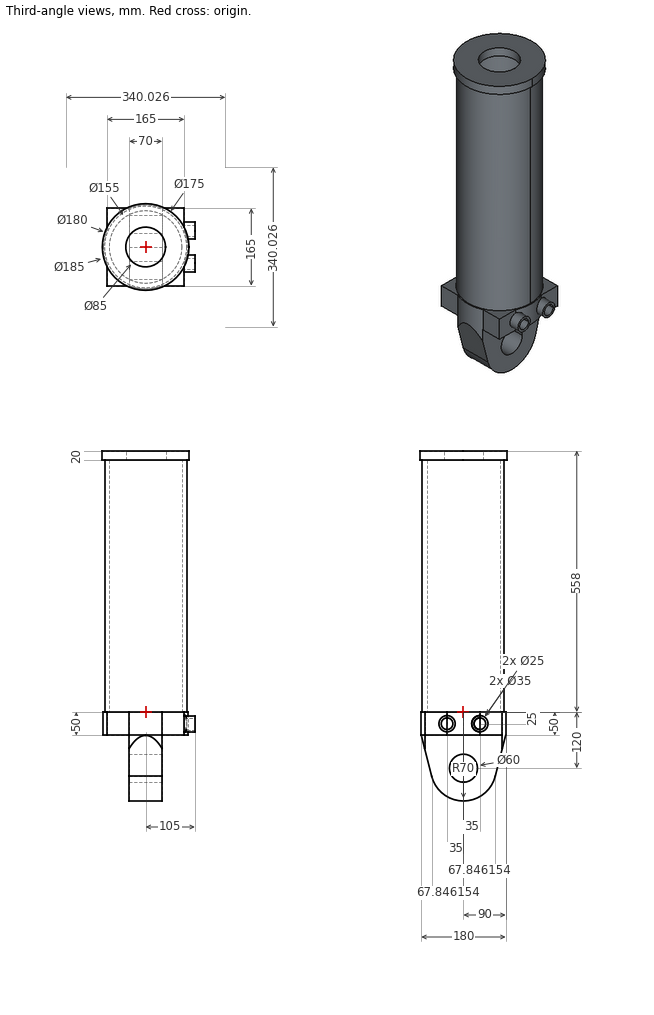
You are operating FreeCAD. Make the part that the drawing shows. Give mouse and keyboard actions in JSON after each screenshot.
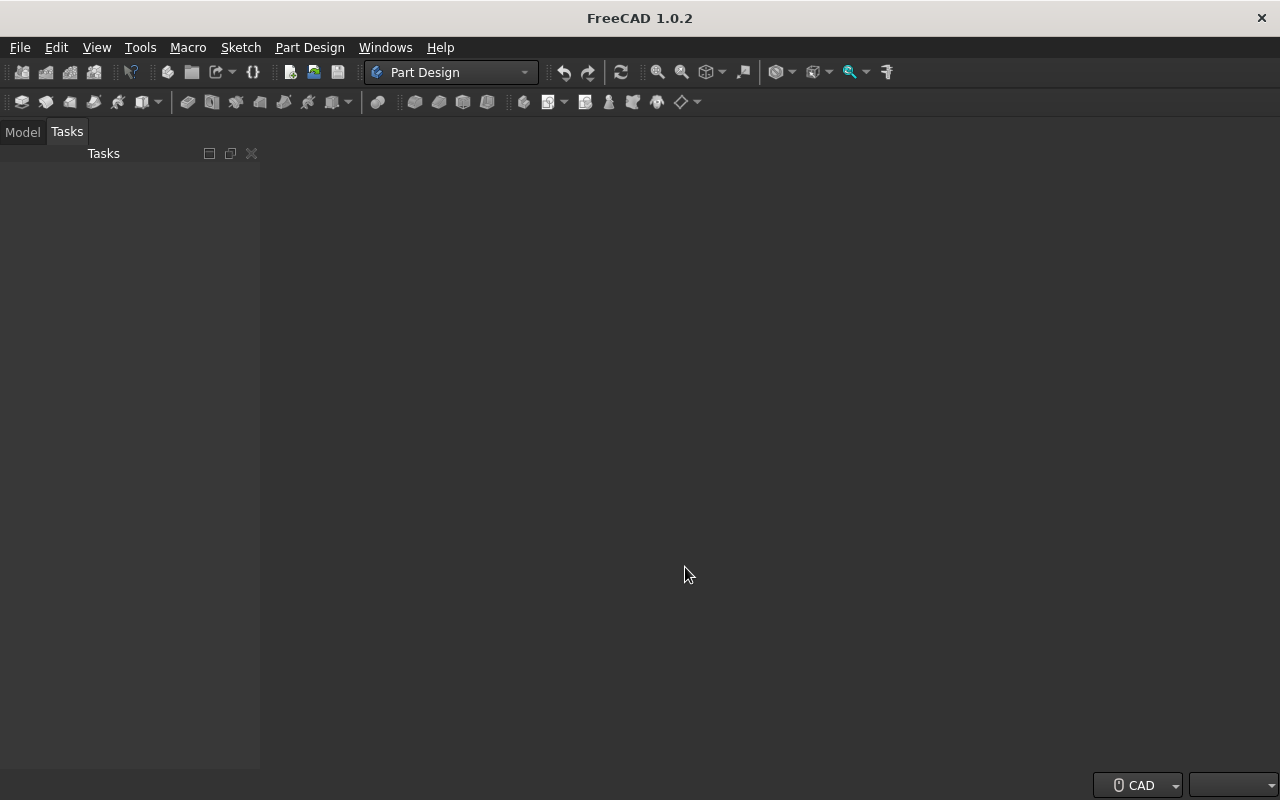
{"action": "key", "text": "ctrl+n"}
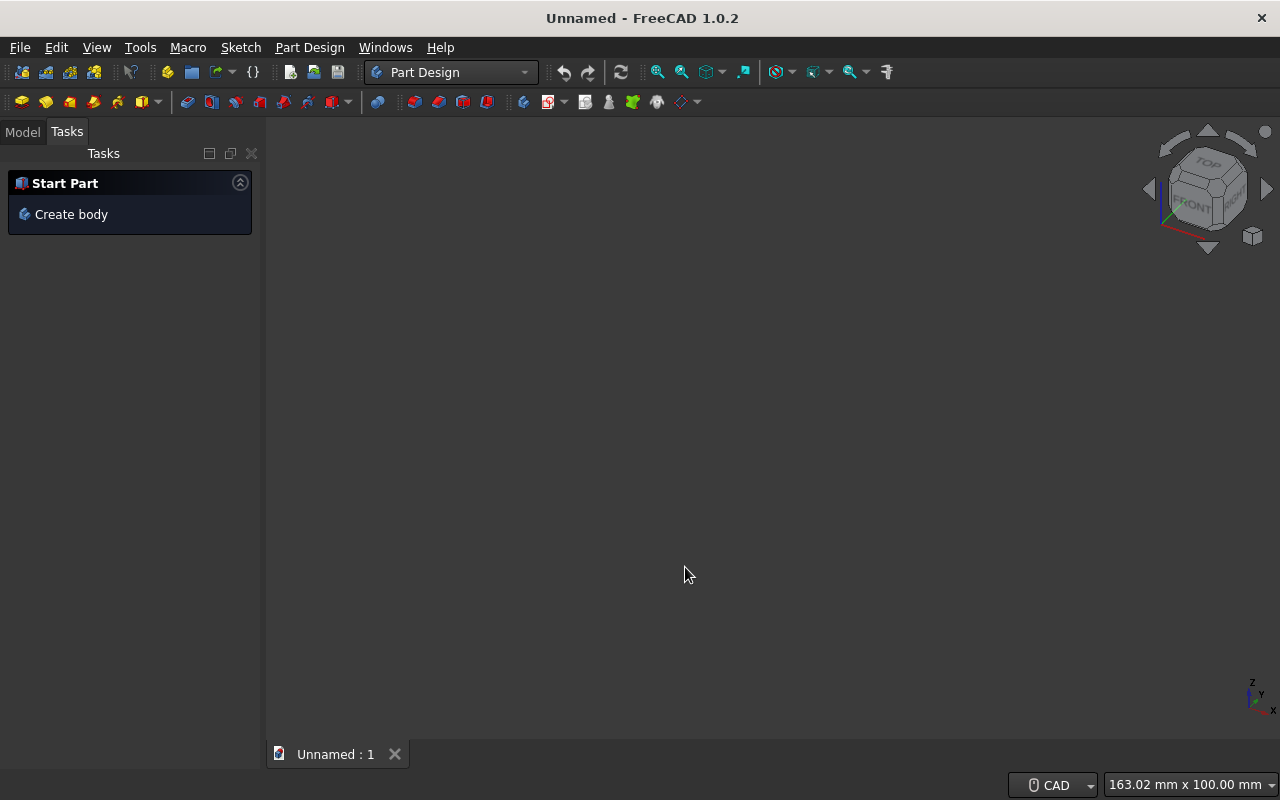
{"action": "left_click", "coordinate": [548, 102]}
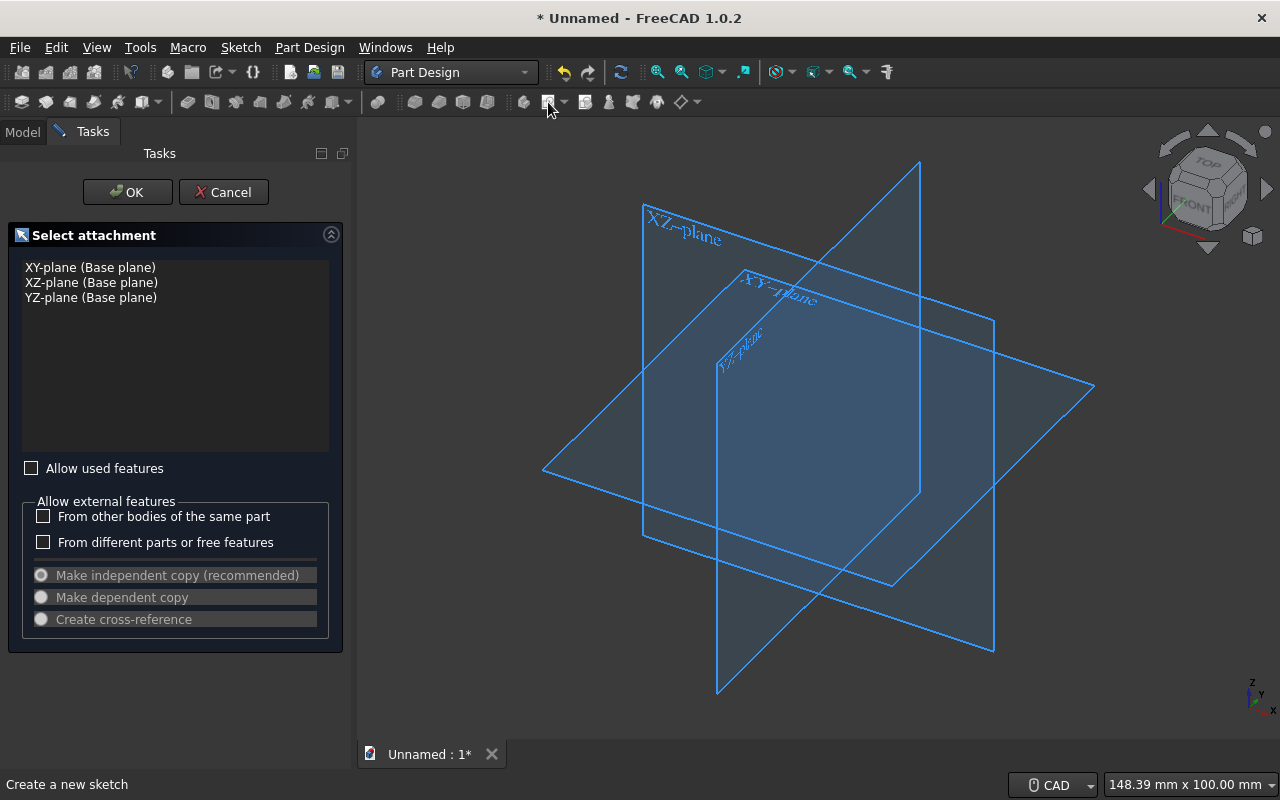
{"action": "left_click", "coordinate": [82, 268]}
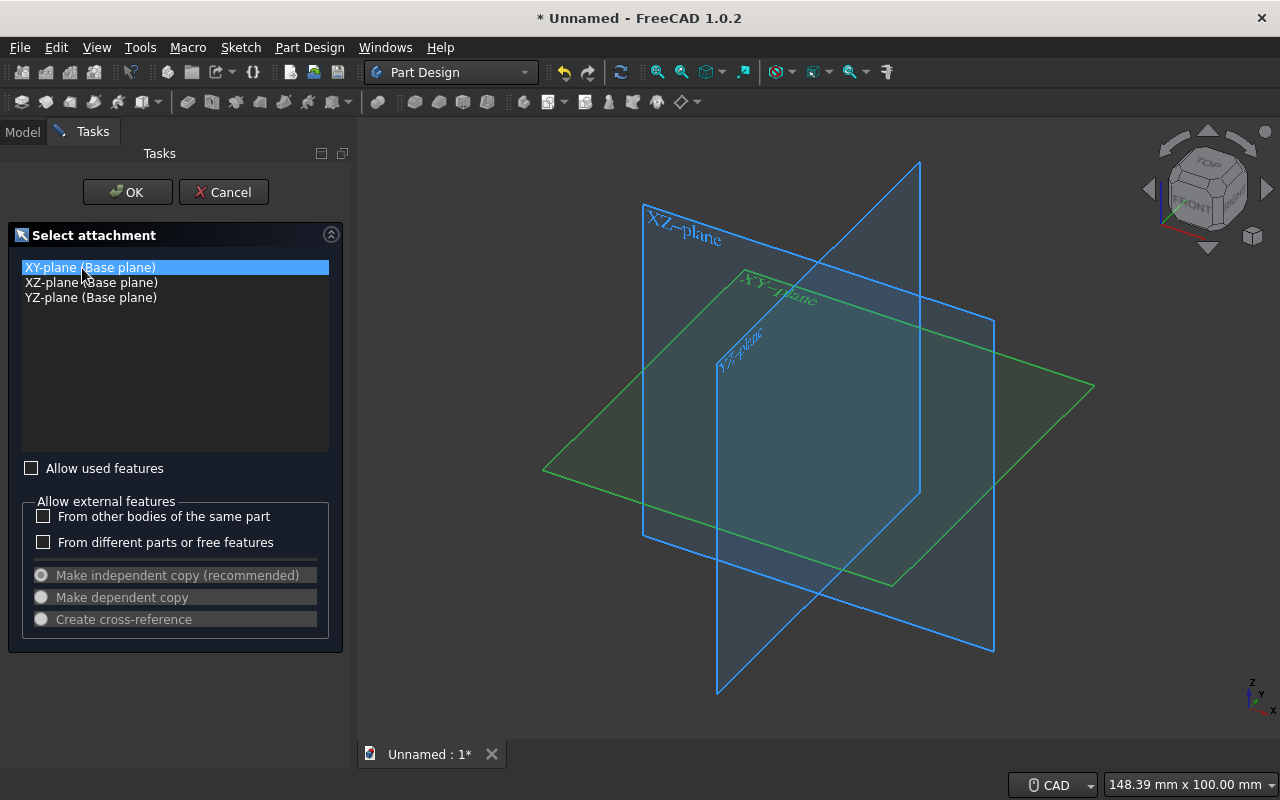
{"action": "left_click", "coordinate": [128, 192]}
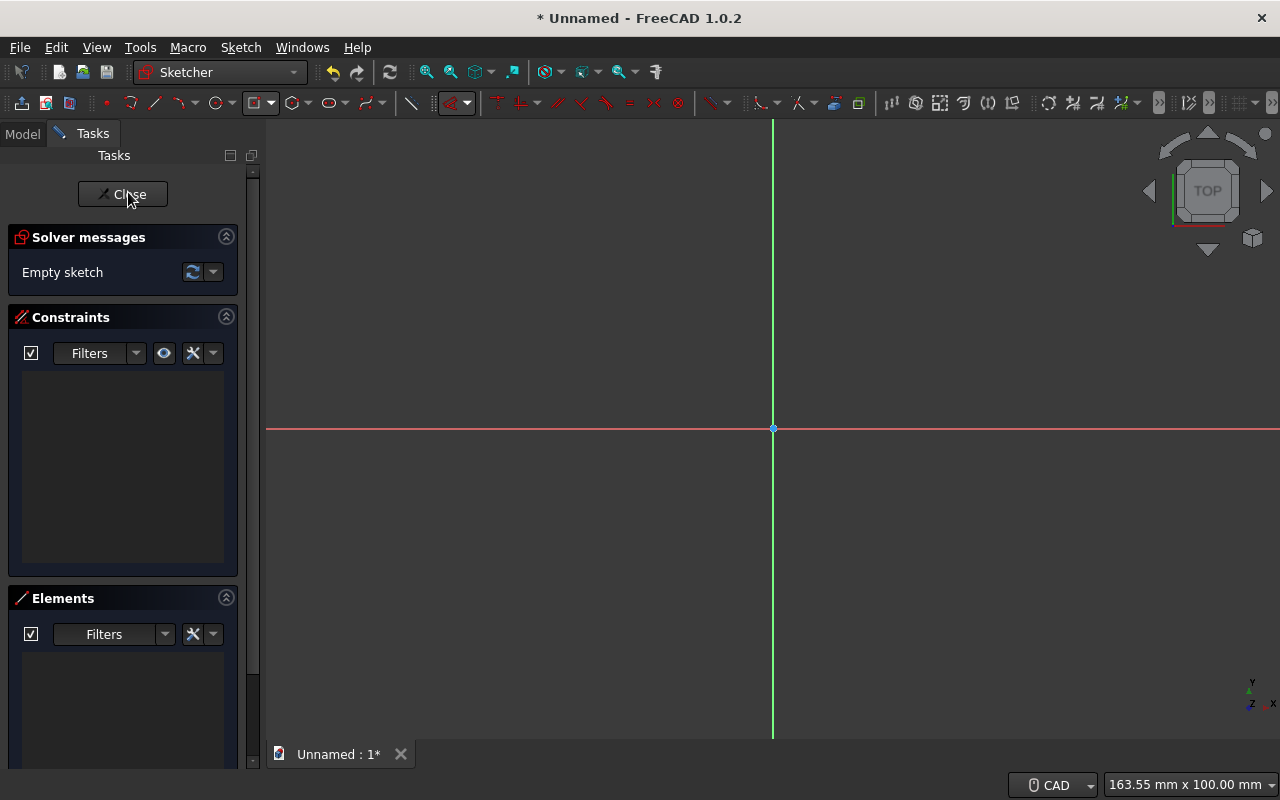
{"action": "scroll", "coordinate": [665, 429], "scroll_direction": "down", "scroll_amount": 5}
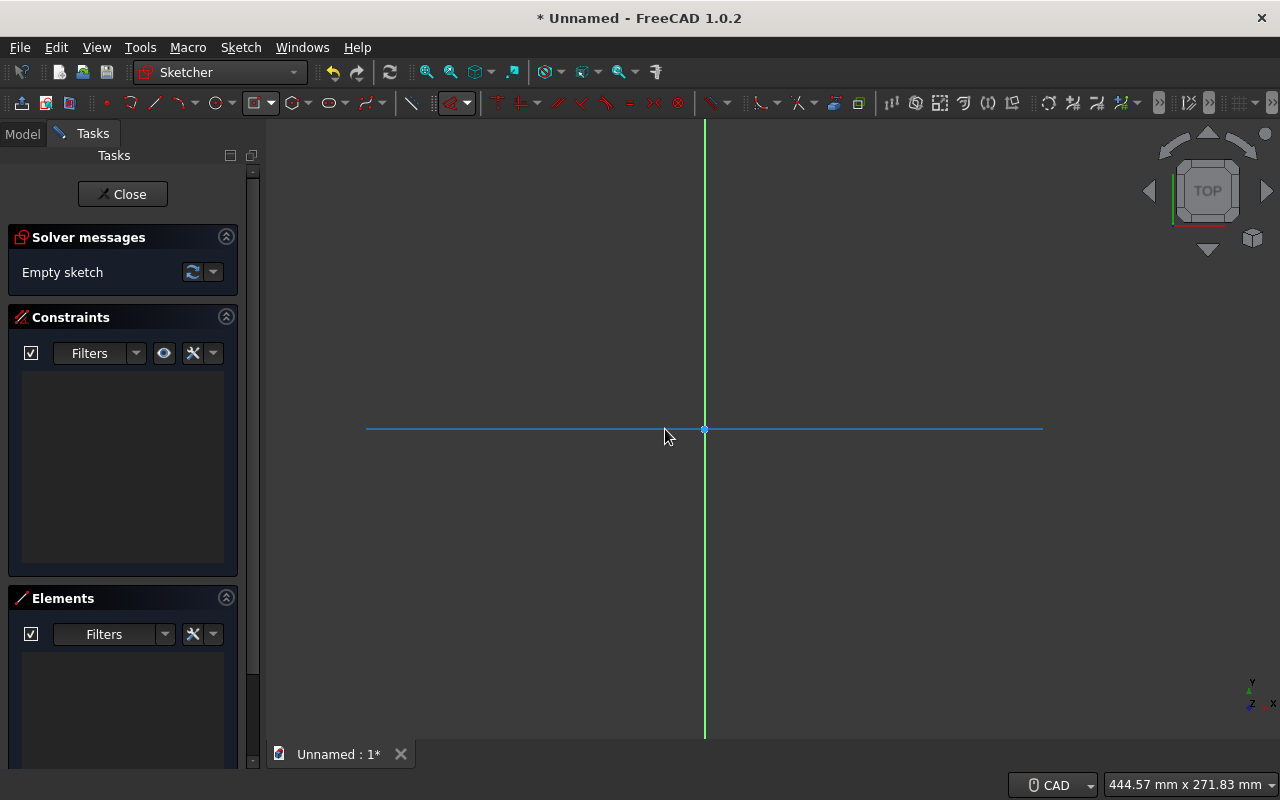
{"action": "left_click", "coordinate": [216, 104]}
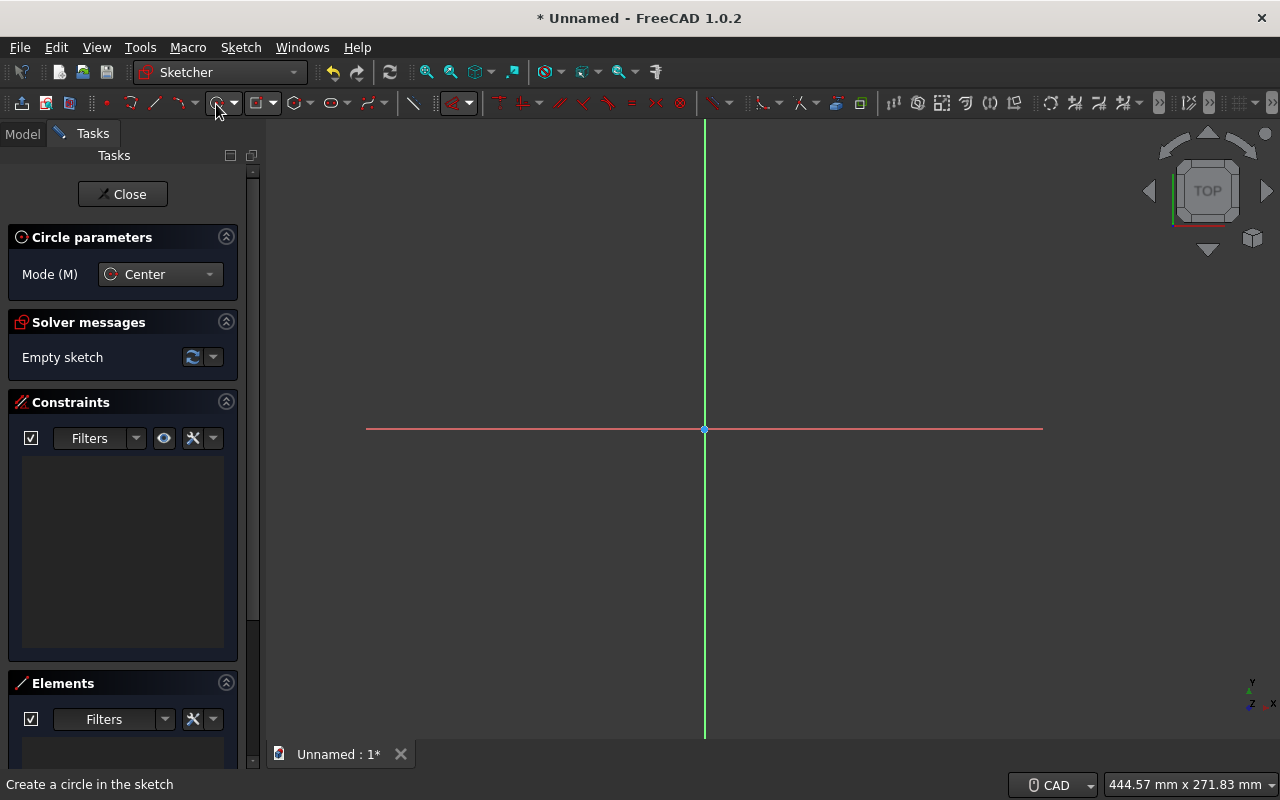
{"action": "left_click", "coordinate": [705, 429]}
{"action": "left_click", "coordinate": [846, 288]}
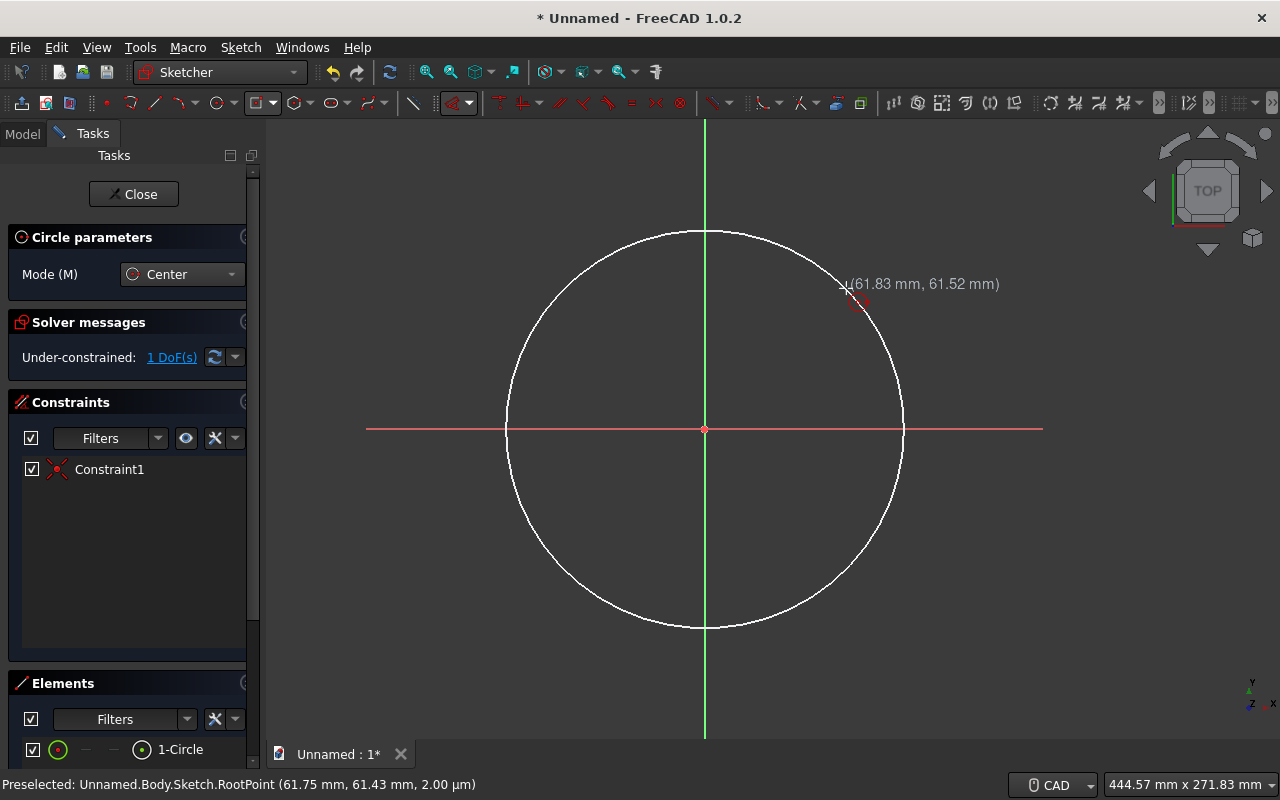
{"action": "left_click", "coordinate": [705, 429]}
{"action": "left_click", "coordinate": [830, 304]}
{"action": "key", "text": "Escape"}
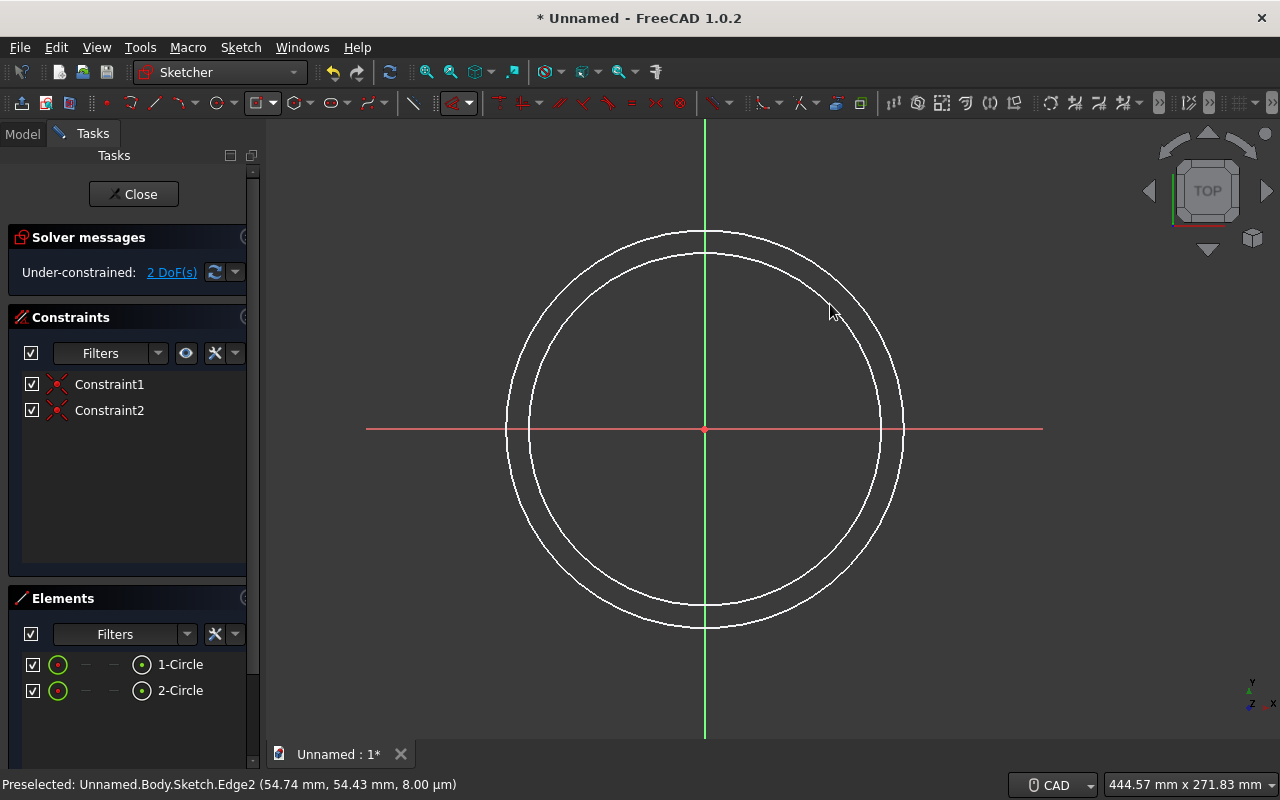
{"action": "key", "text": "d"}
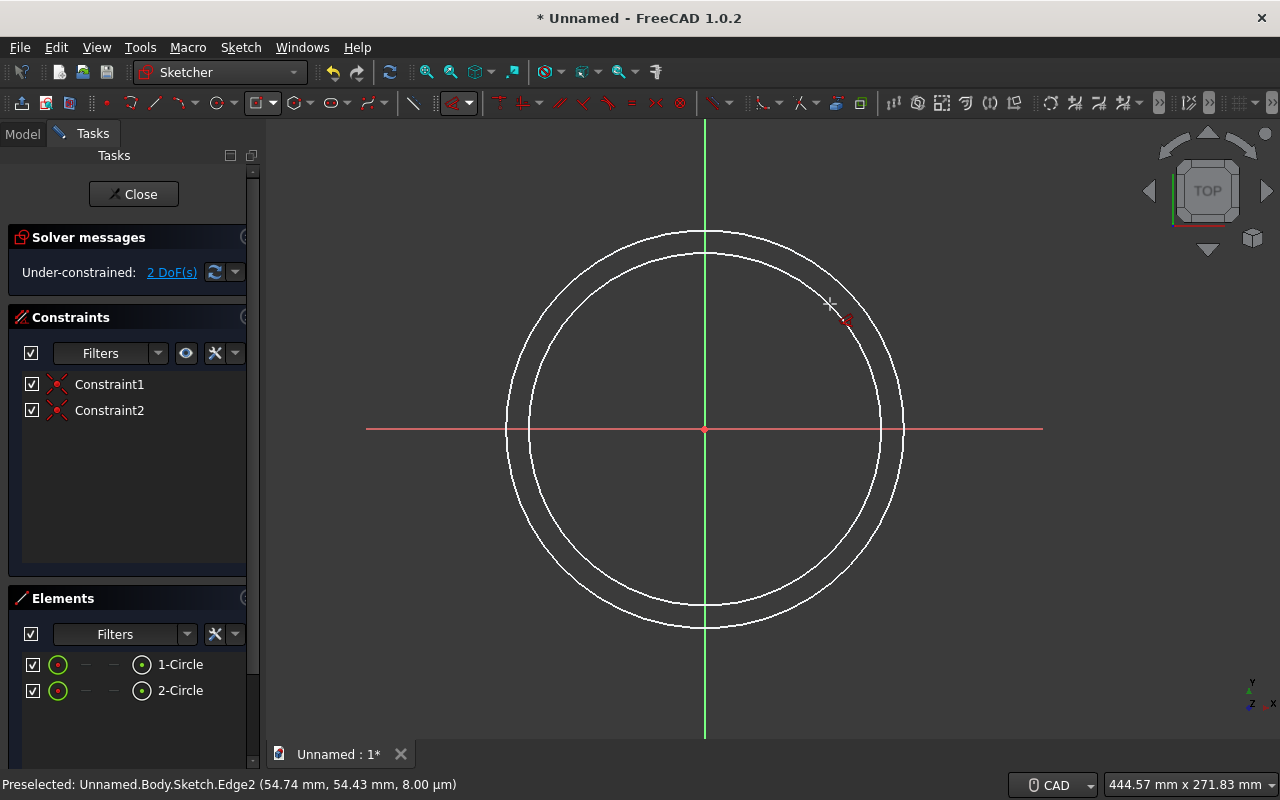
{"action": "left_click", "coordinate": [845, 288]}
{"action": "left_click", "coordinate": [868, 265]}